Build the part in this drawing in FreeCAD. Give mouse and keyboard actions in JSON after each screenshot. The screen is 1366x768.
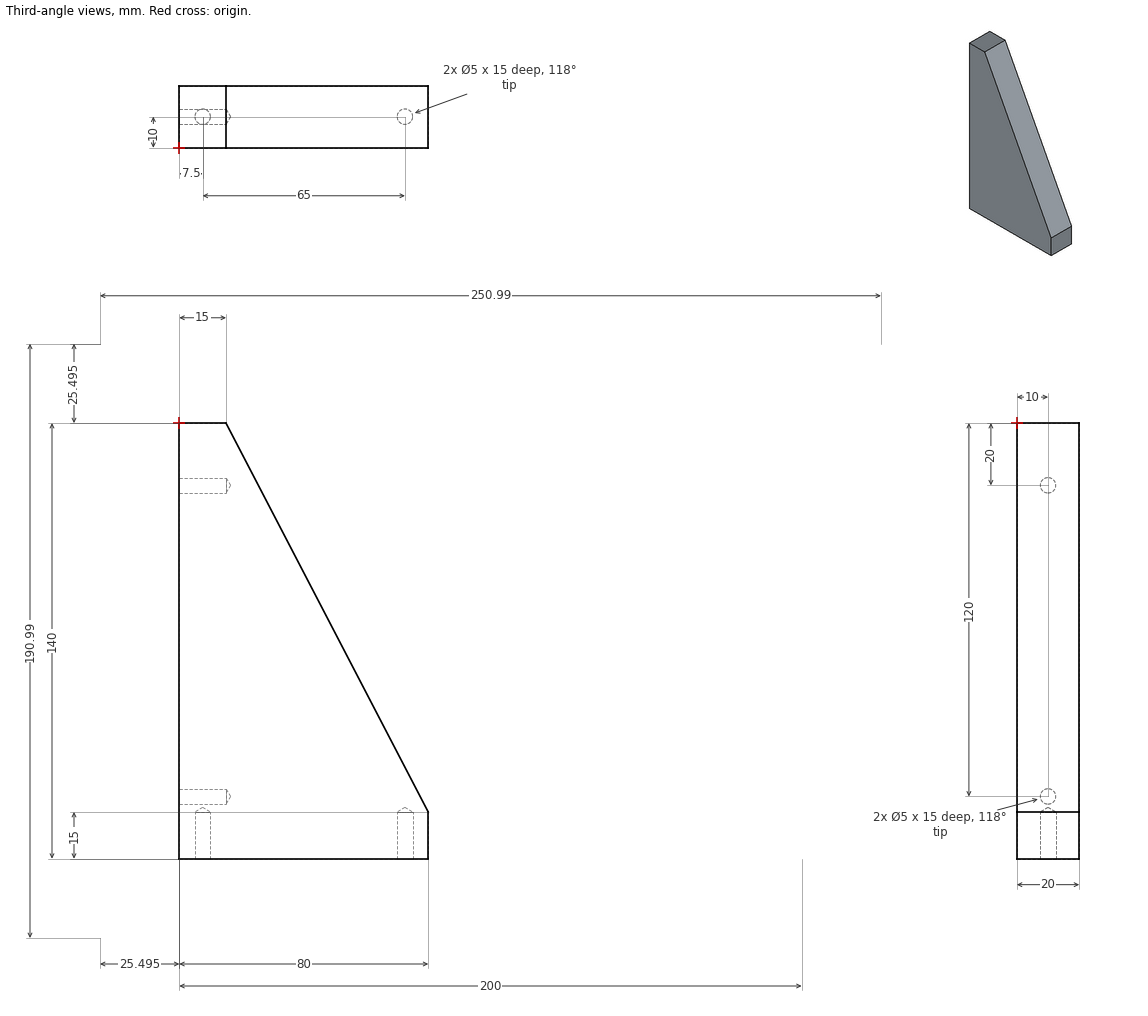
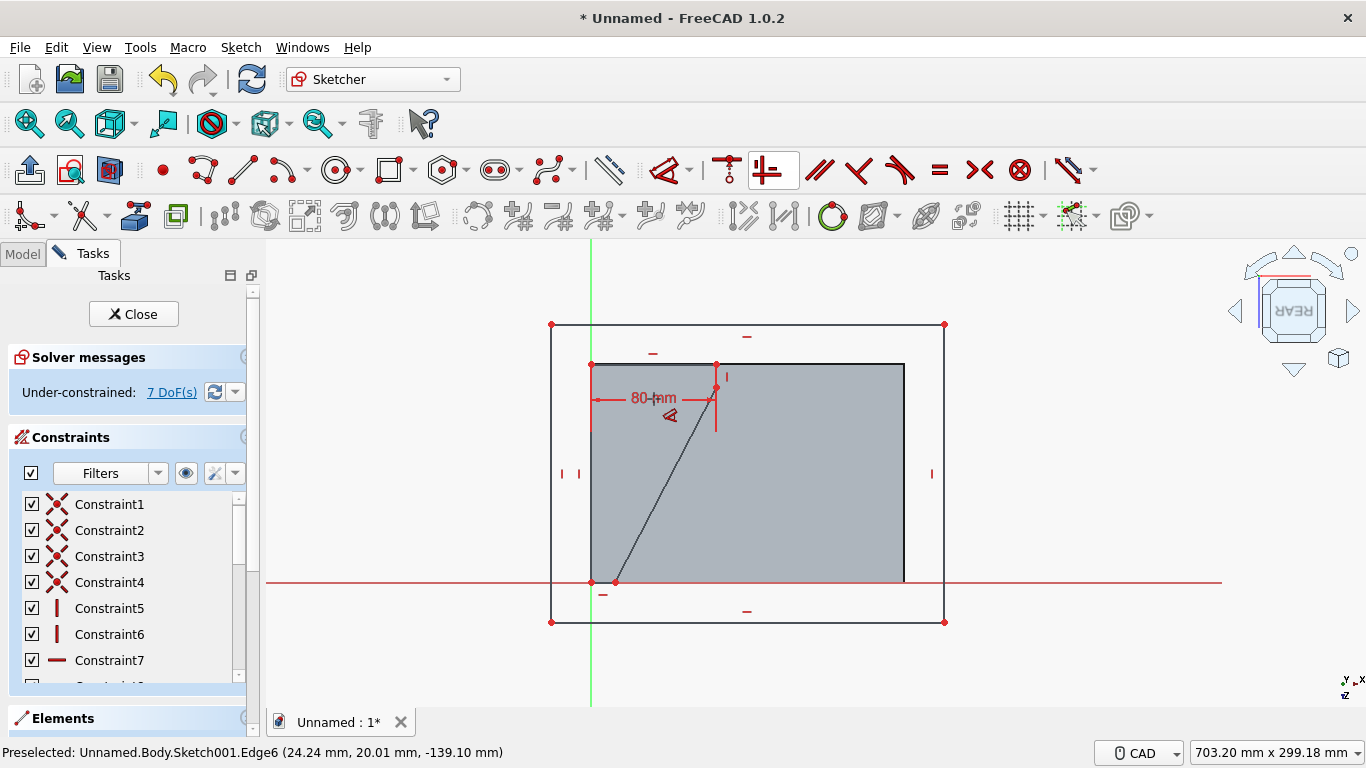
{"action": "scroll", "coordinate": [716, 374], "scroll_direction": "up", "scroll_amount": 3}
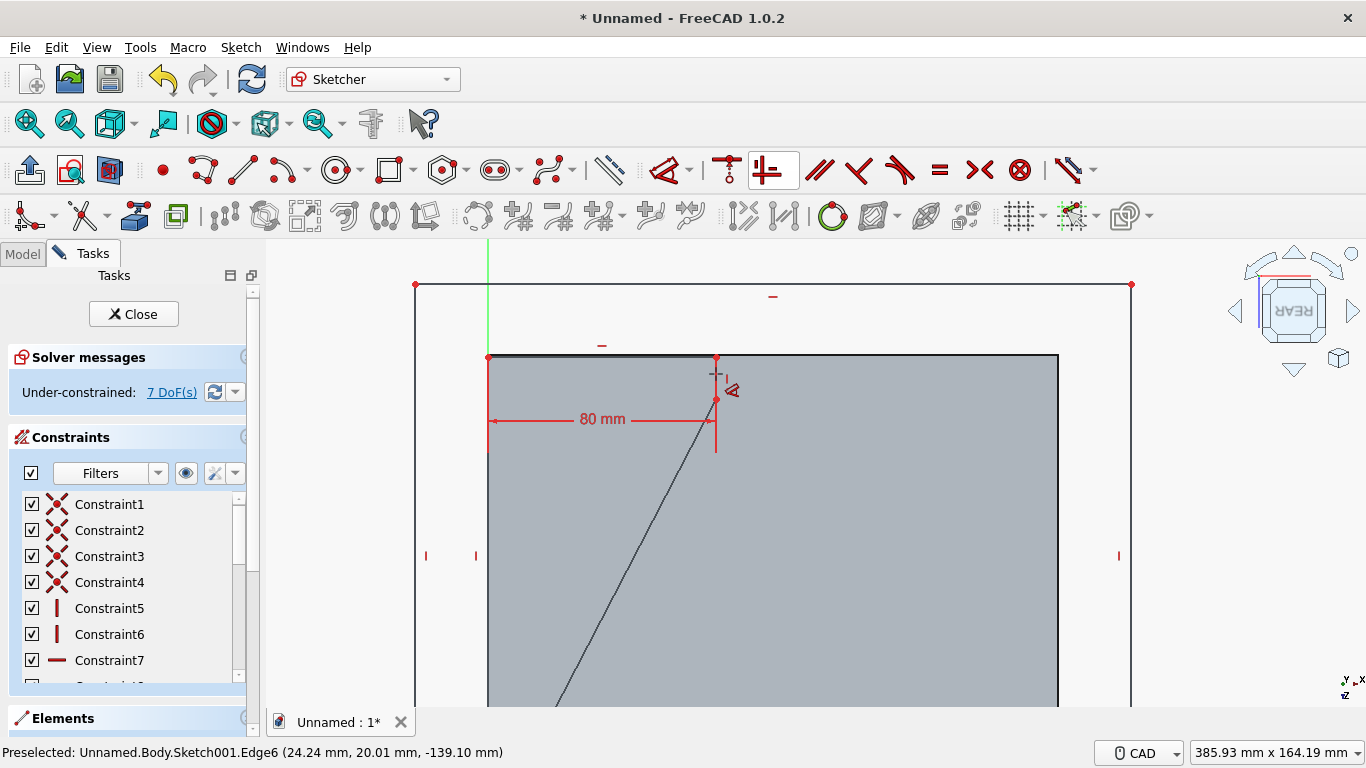
{"action": "left_click", "coordinate": [716, 374]}
{"action": "left_click", "coordinate": [682, 378]}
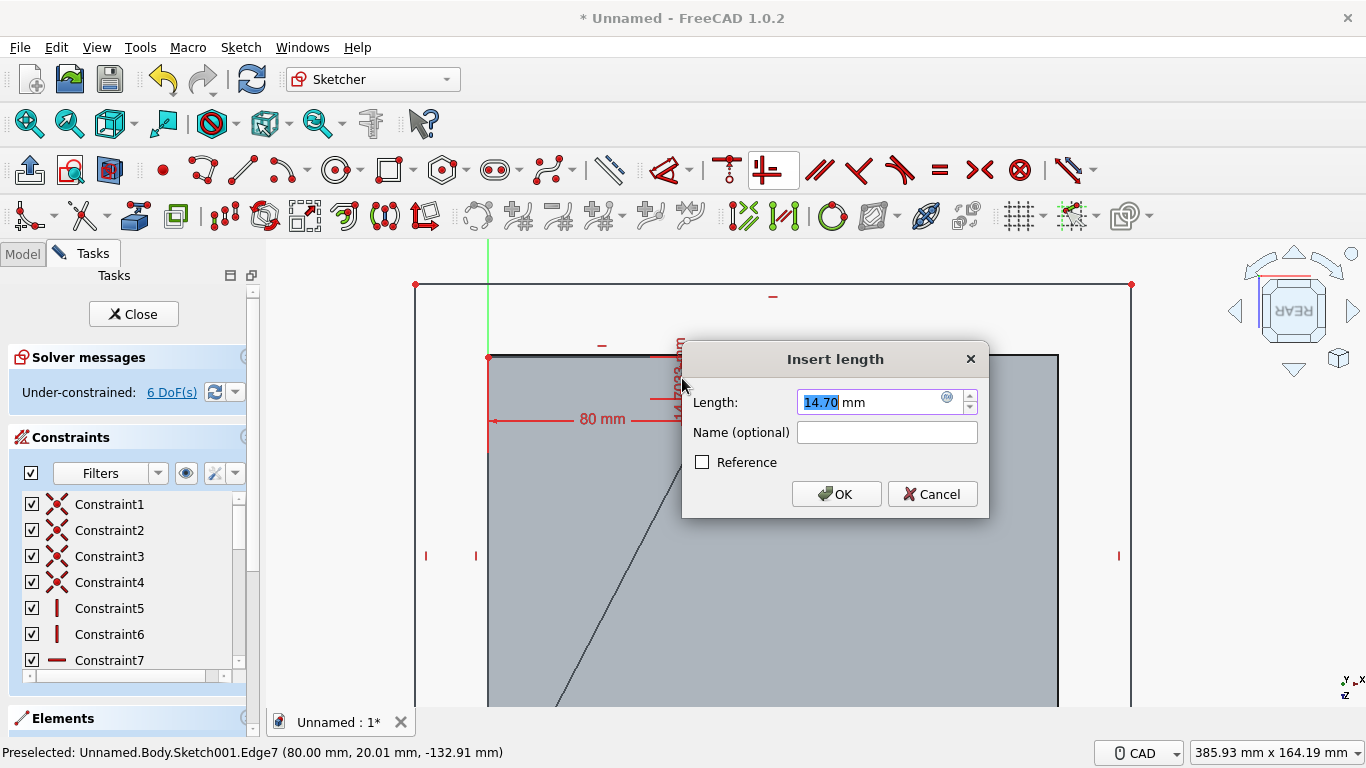
{"action": "type", "text": "15"}
{"action": "key", "text": "Return"}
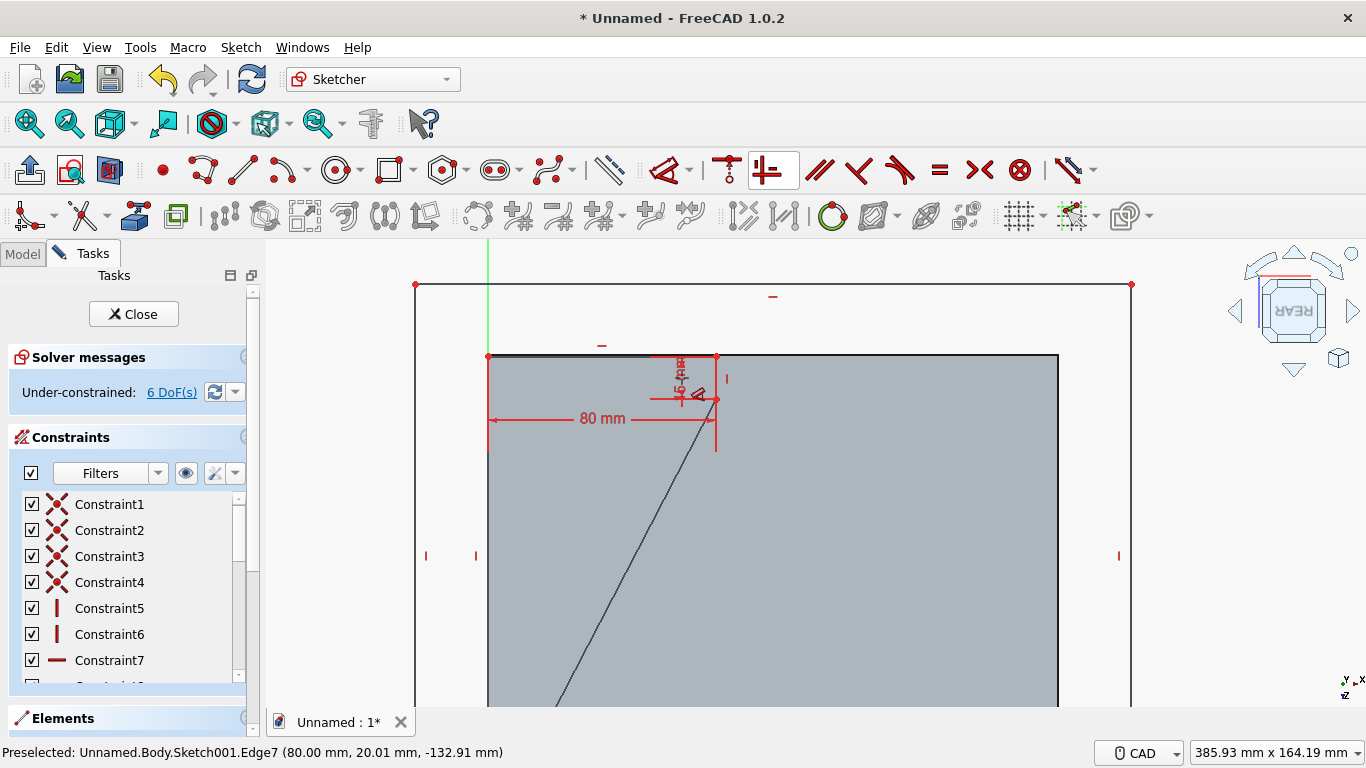
{"action": "scroll", "coordinate": [716, 374], "scroll_direction": "down", "scroll_amount": 3}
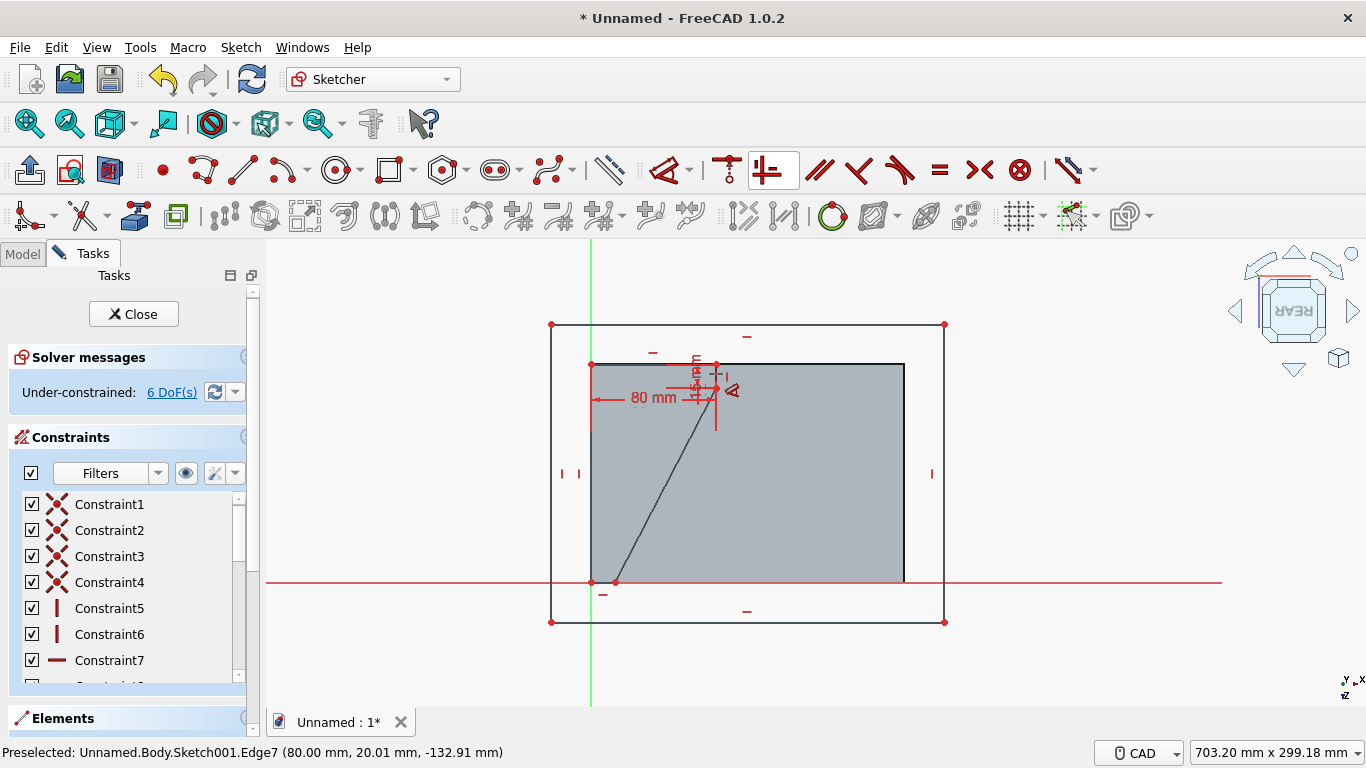
{"action": "scroll", "coordinate": [608, 583], "scroll_direction": "up", "scroll_amount": 4}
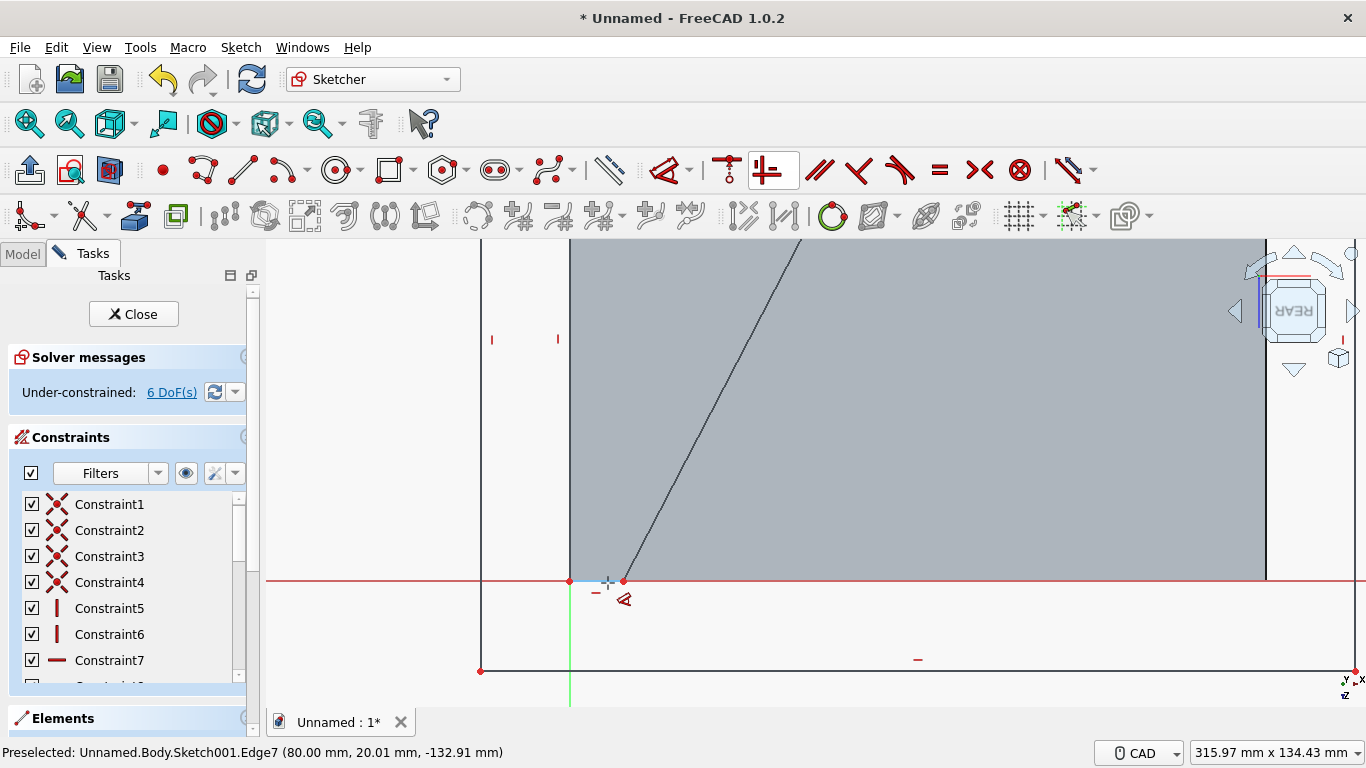
{"action": "left_click", "coordinate": [607, 581]}
{"action": "left_click", "coordinate": [597, 615]}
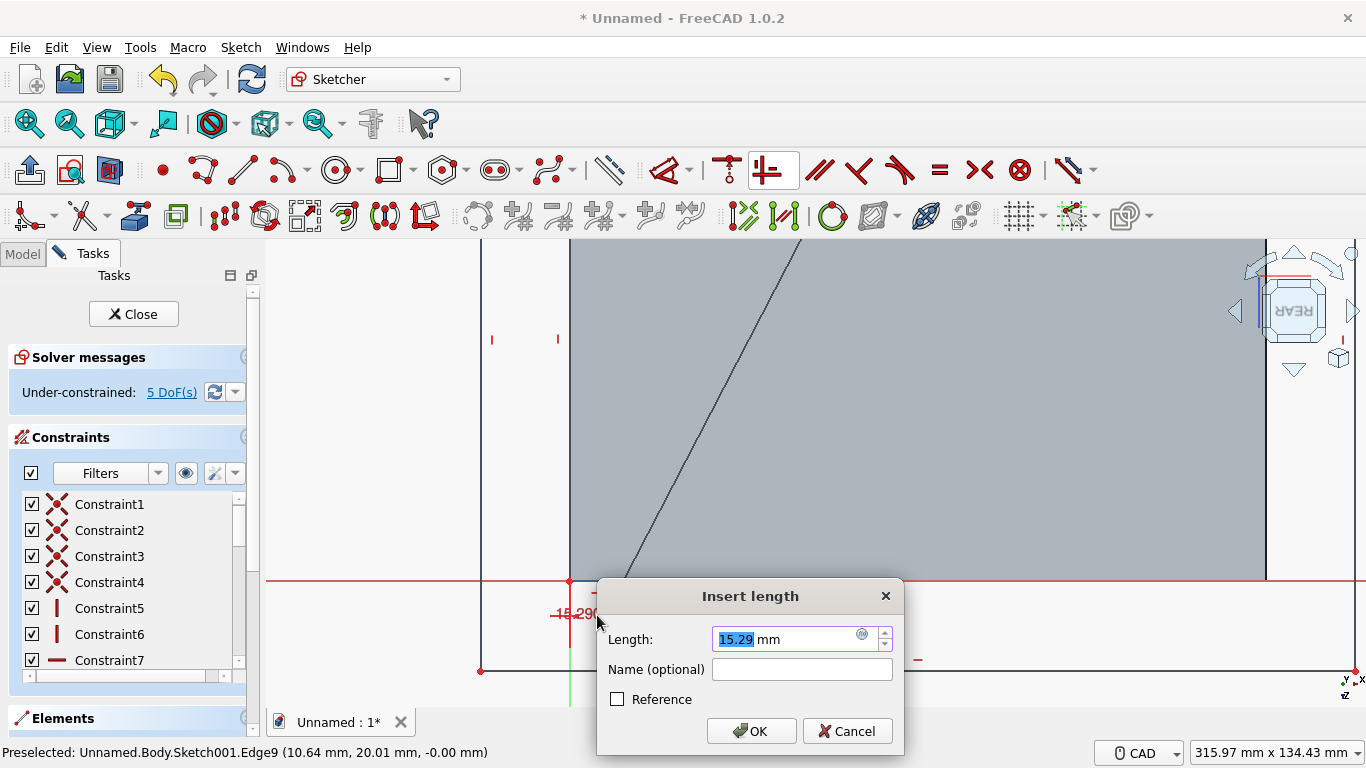
{"action": "type", "text": "15"}
{"action": "key", "text": "Return"}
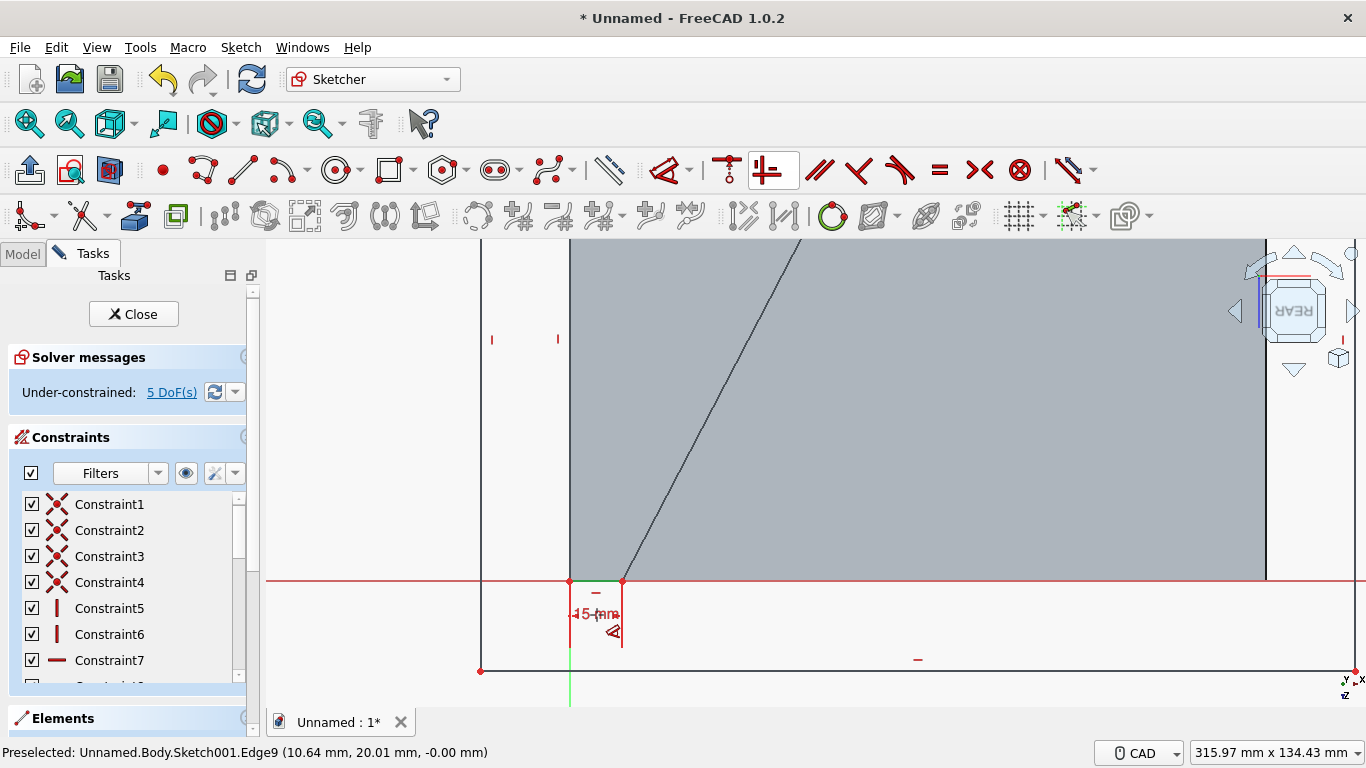
{"action": "left_click", "coordinate": [570, 436]}
{"action": "left_click", "coordinate": [536, 424]}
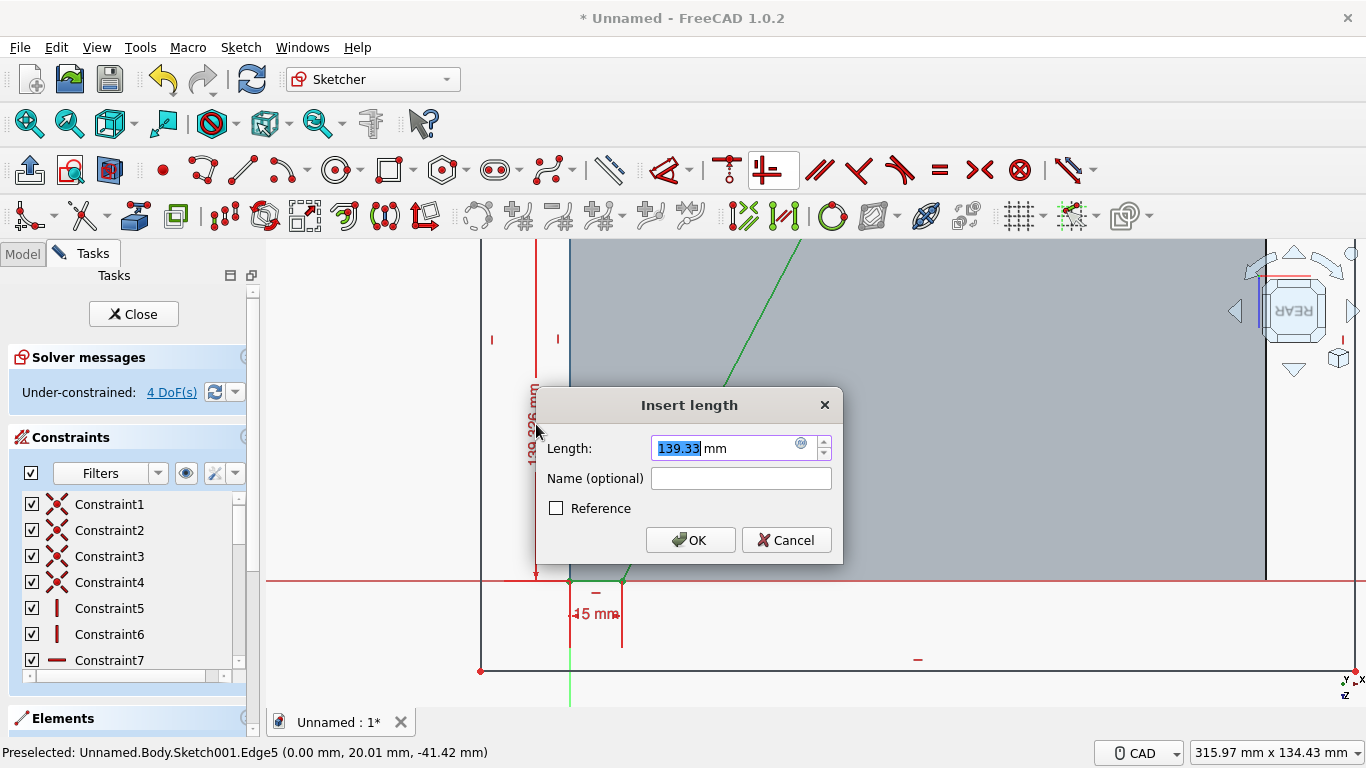
{"action": "type", "text": "140"}
{"action": "key", "text": "Return"}